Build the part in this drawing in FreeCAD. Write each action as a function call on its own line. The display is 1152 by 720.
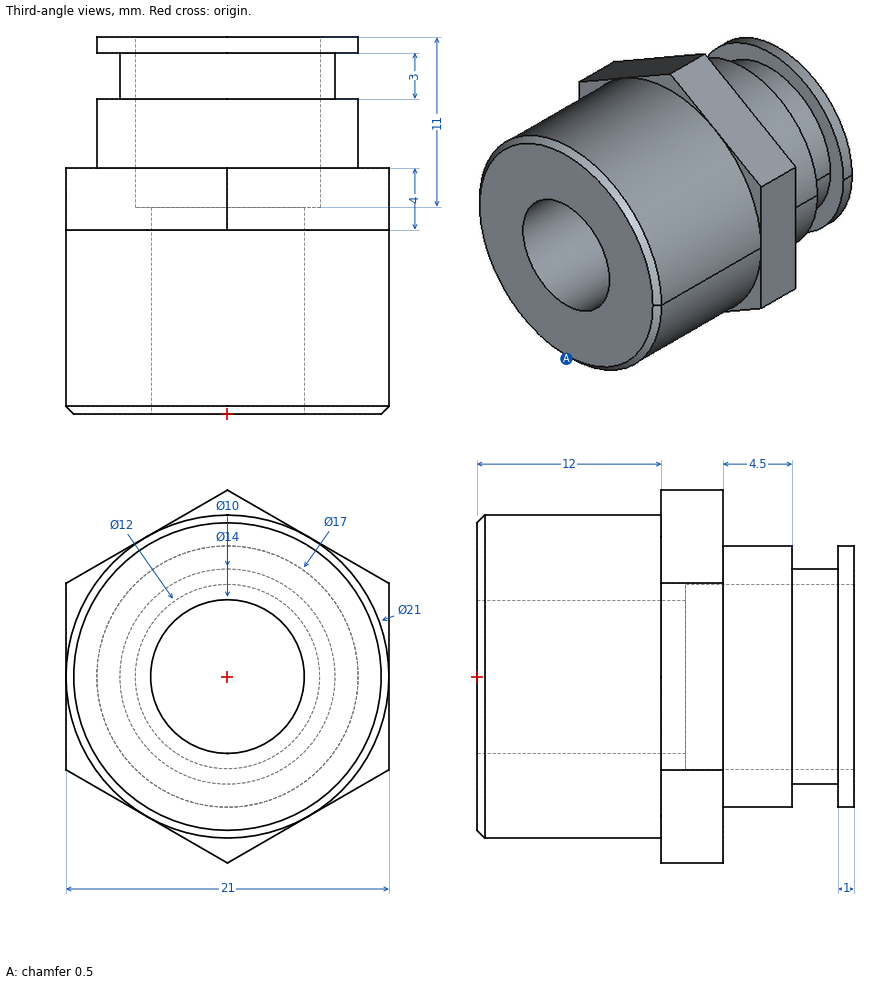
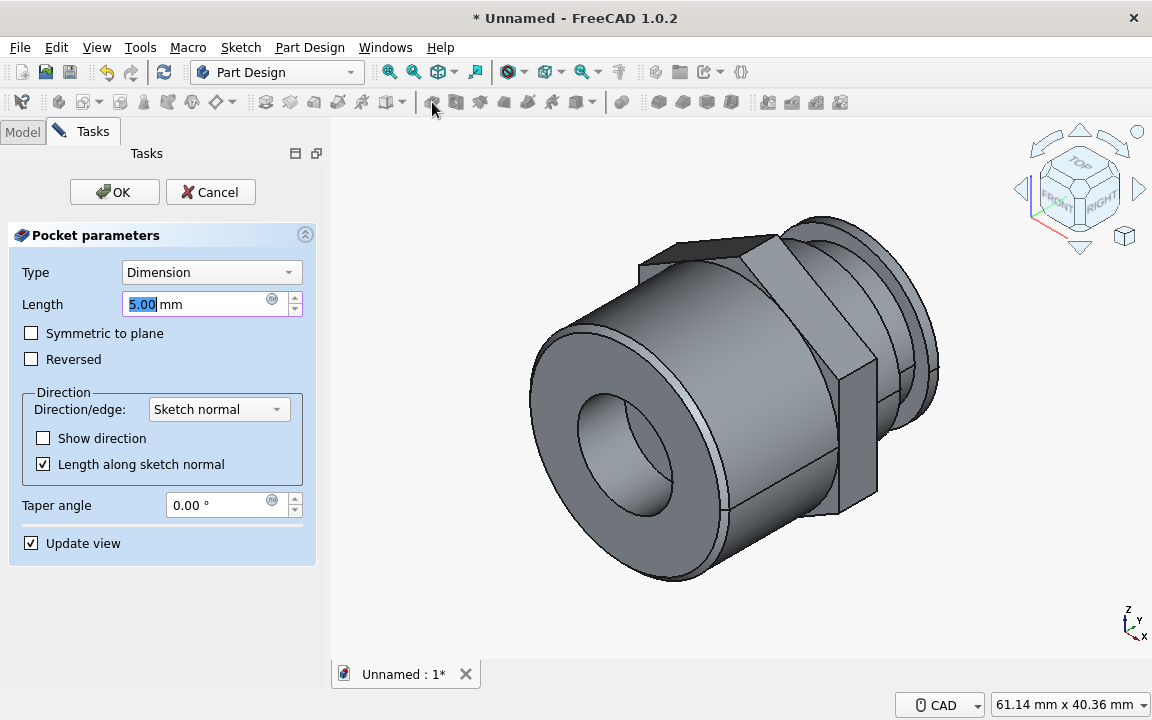
click(212, 272)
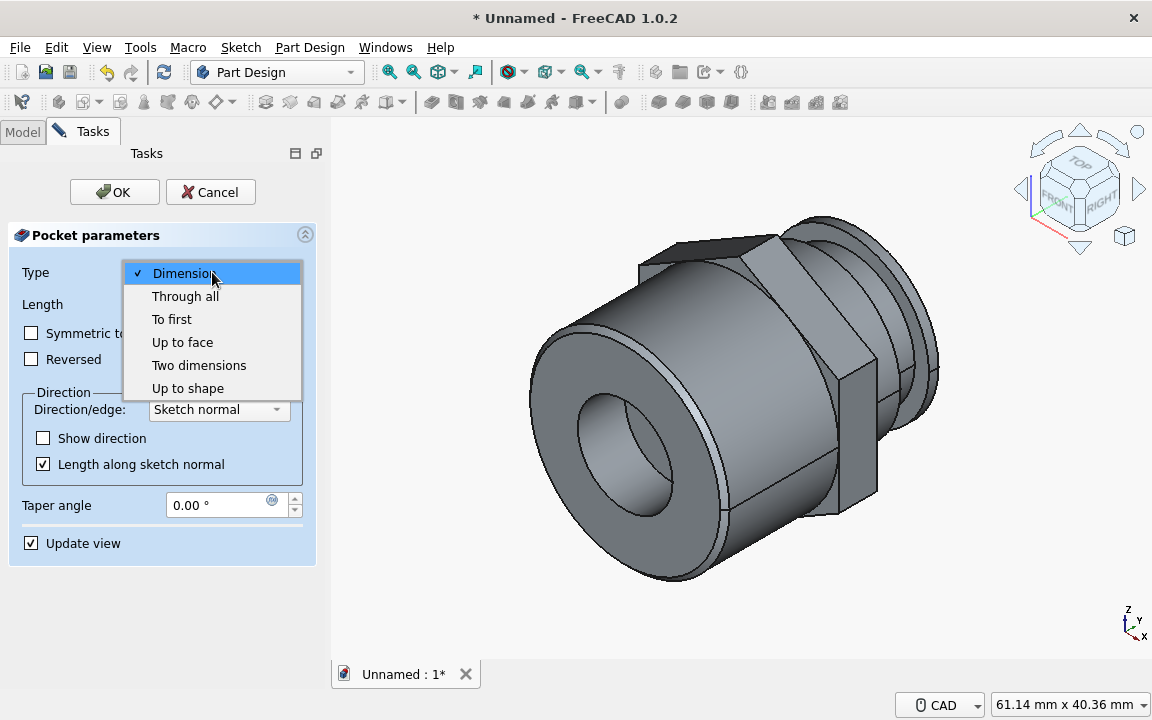
click(212, 296)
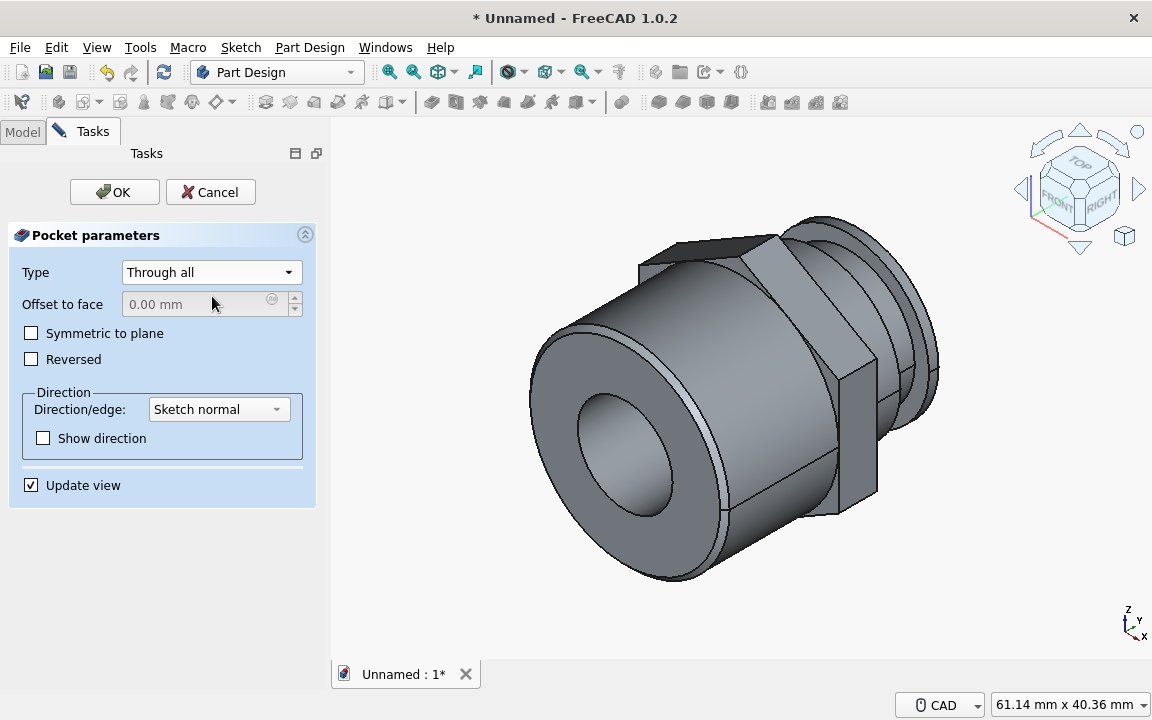
click(115, 192)